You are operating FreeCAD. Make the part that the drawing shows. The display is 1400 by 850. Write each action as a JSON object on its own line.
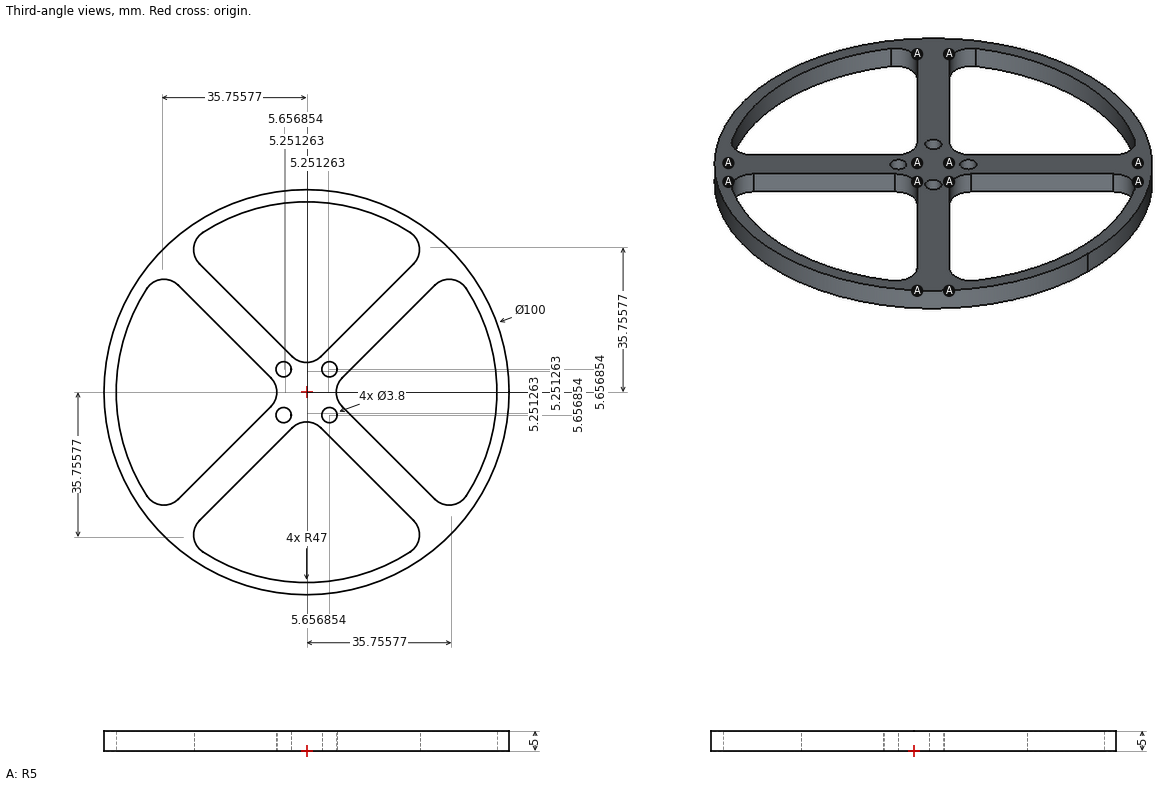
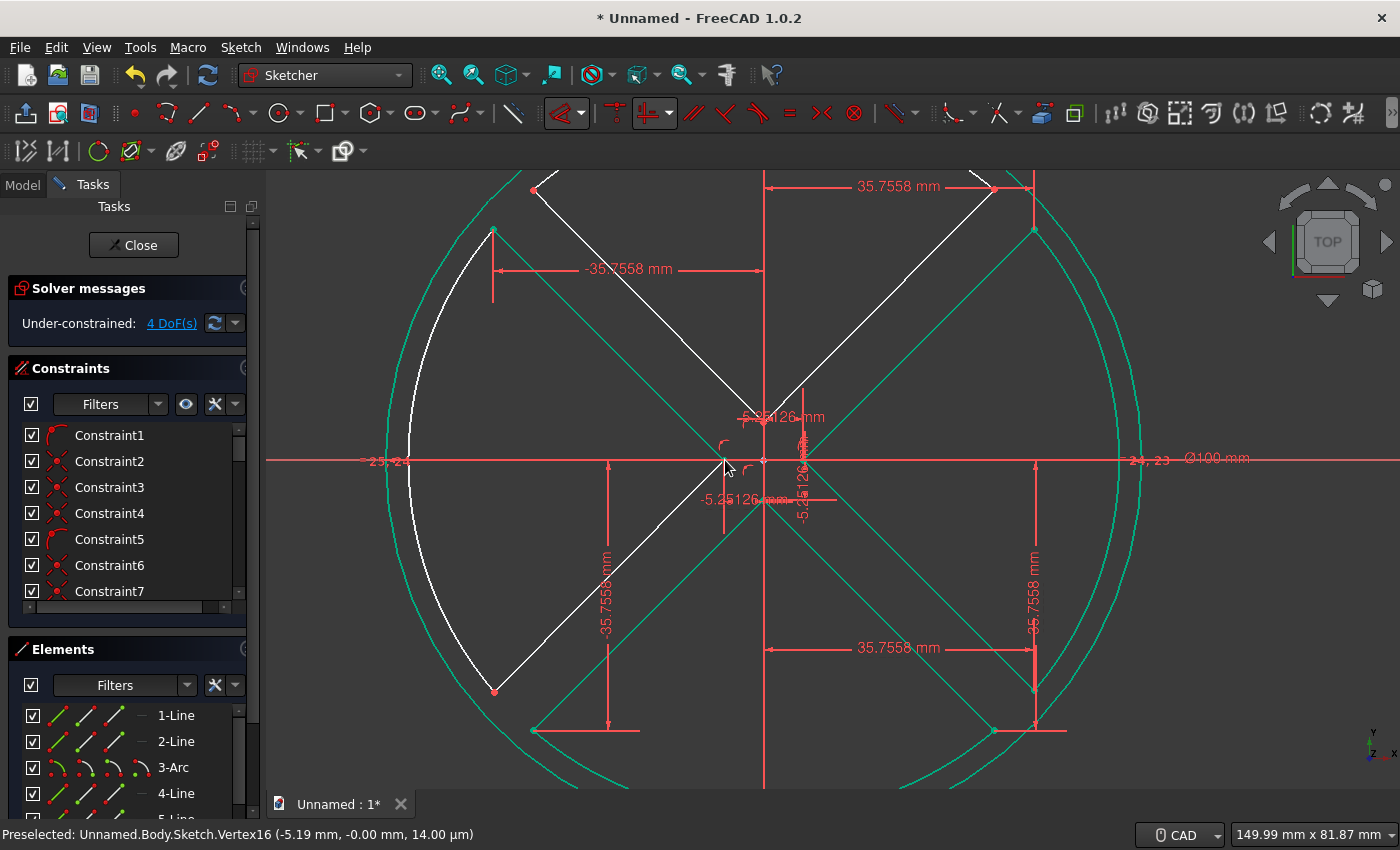
{"action": "left_click", "coordinate": [494, 692]}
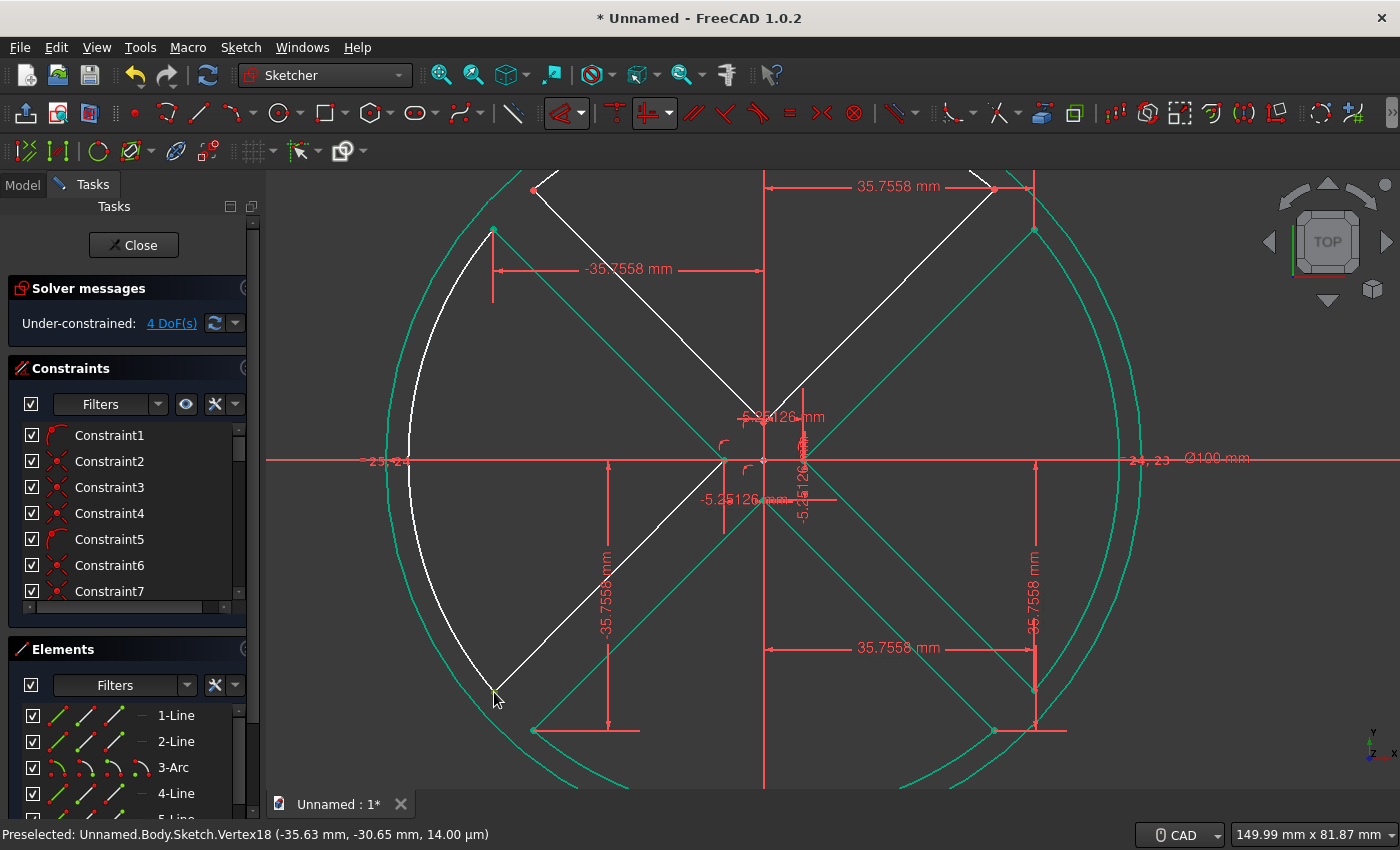
{"action": "key", "text": "l"}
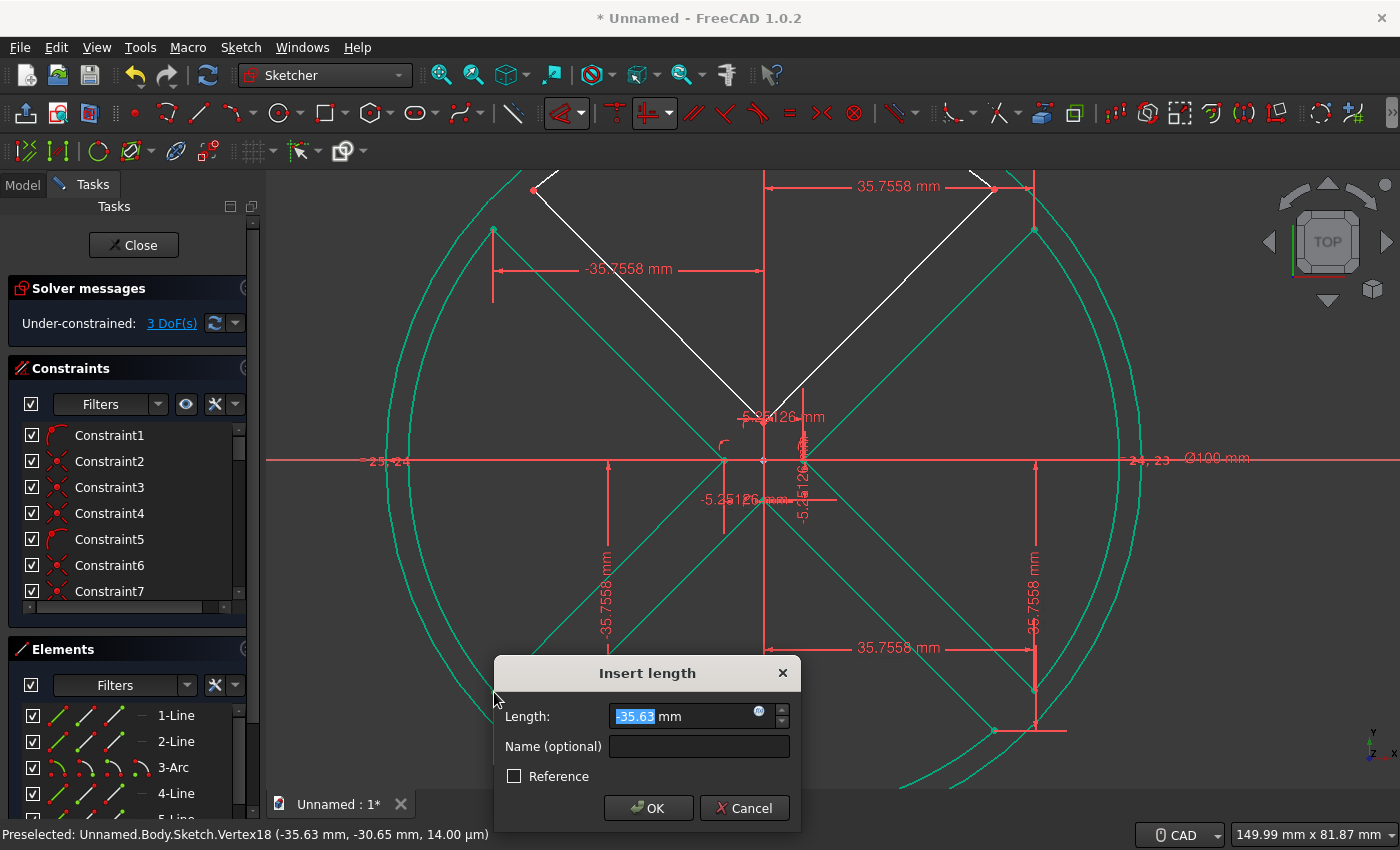
{"action": "type", "text": "-35.75577"}
{"action": "key", "text": "Return"}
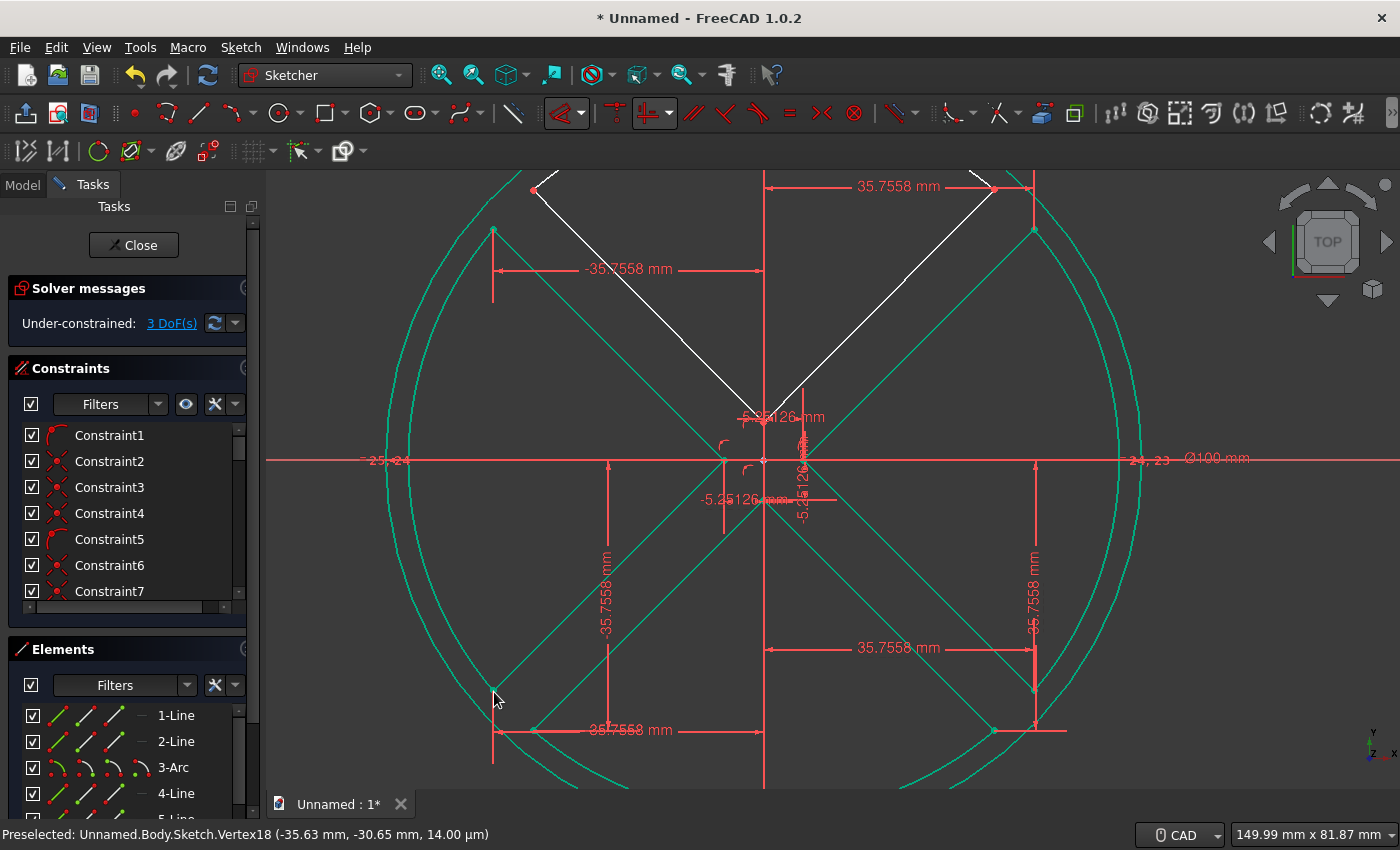
{"action": "scroll", "coordinate": [765, 503], "scroll_direction": "down", "scroll_amount": 3}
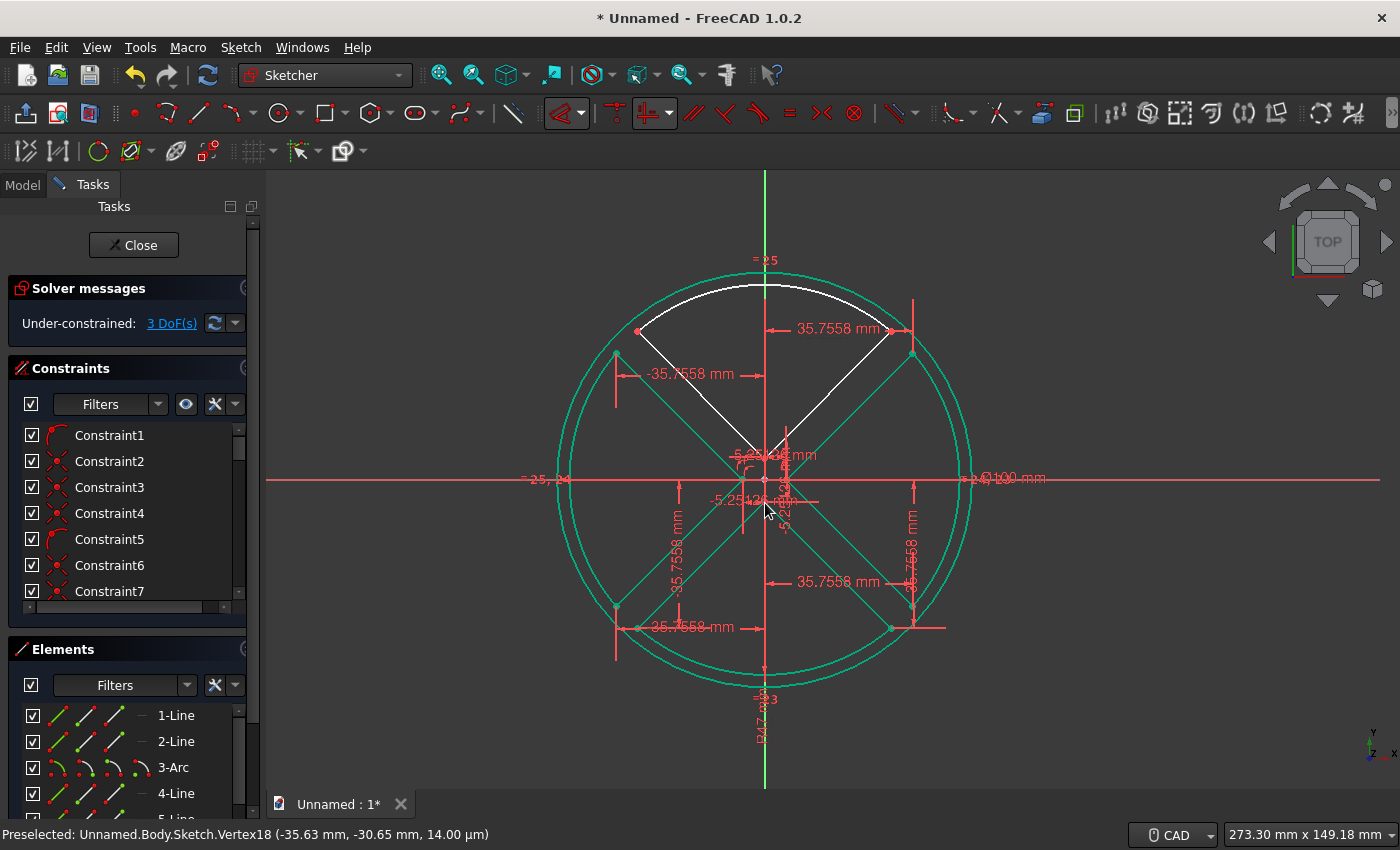
{"action": "left_click", "coordinate": [891, 331]}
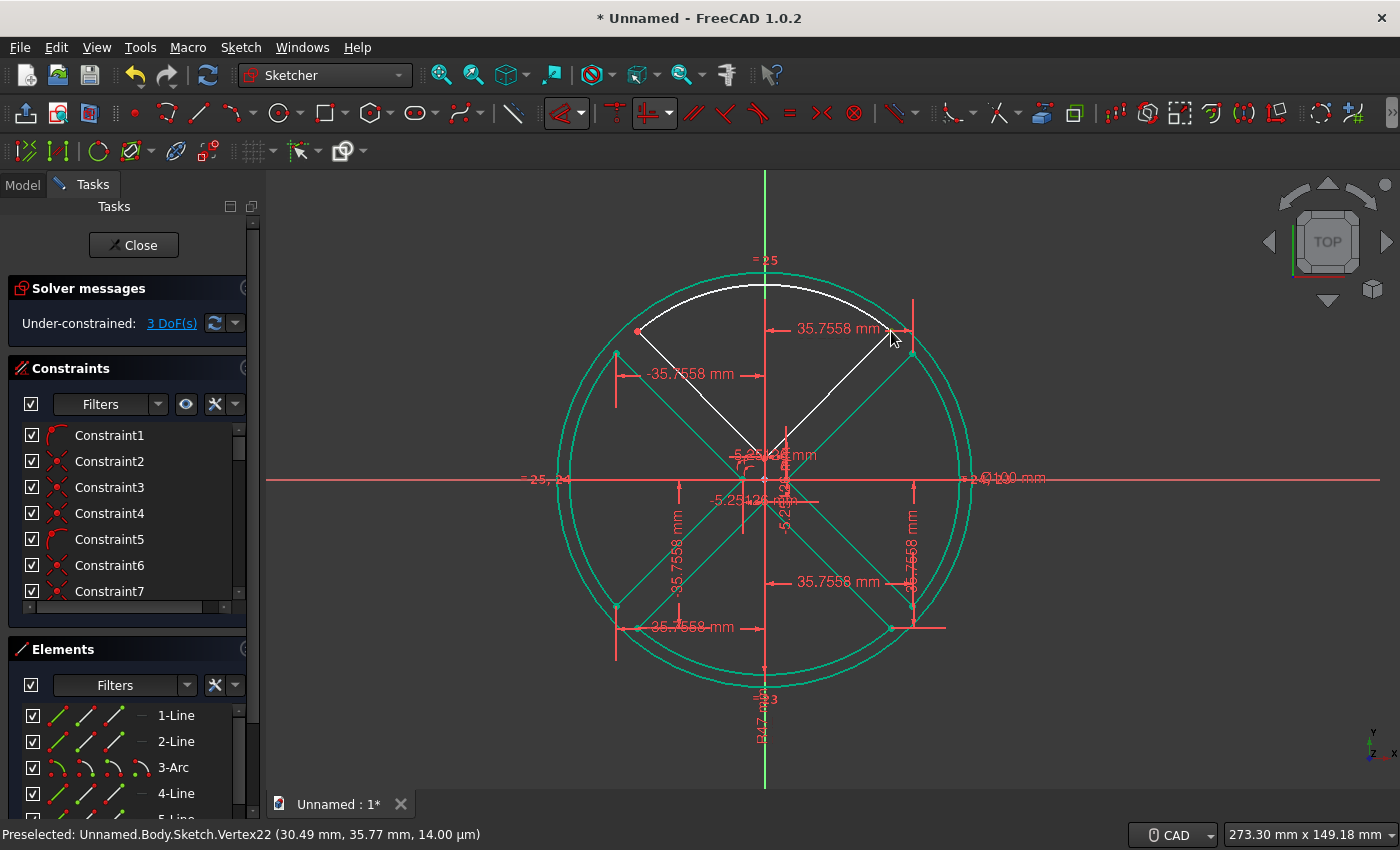
{"action": "left_click", "coordinate": [584, 114]}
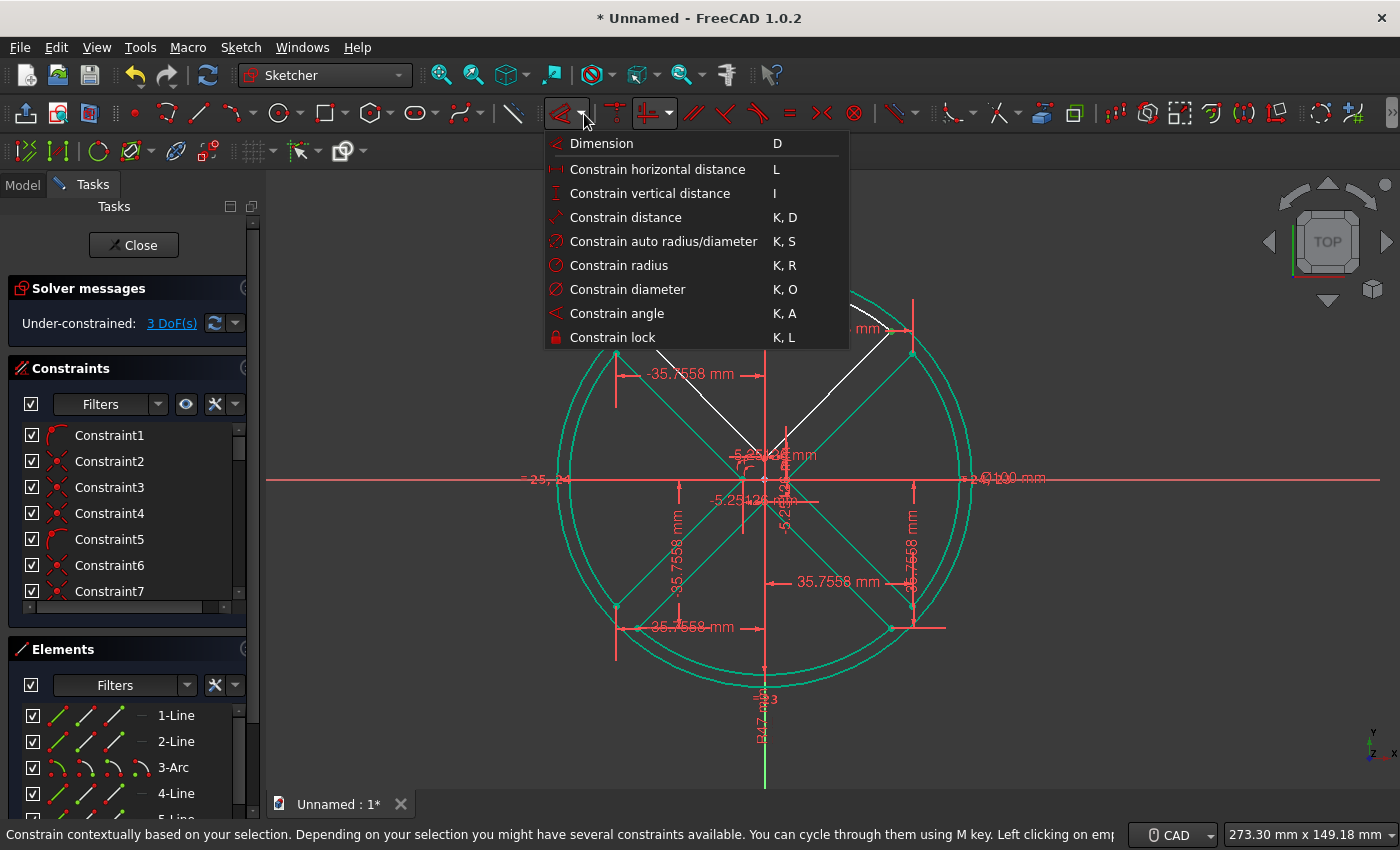
{"action": "left_click", "coordinate": [697, 193]}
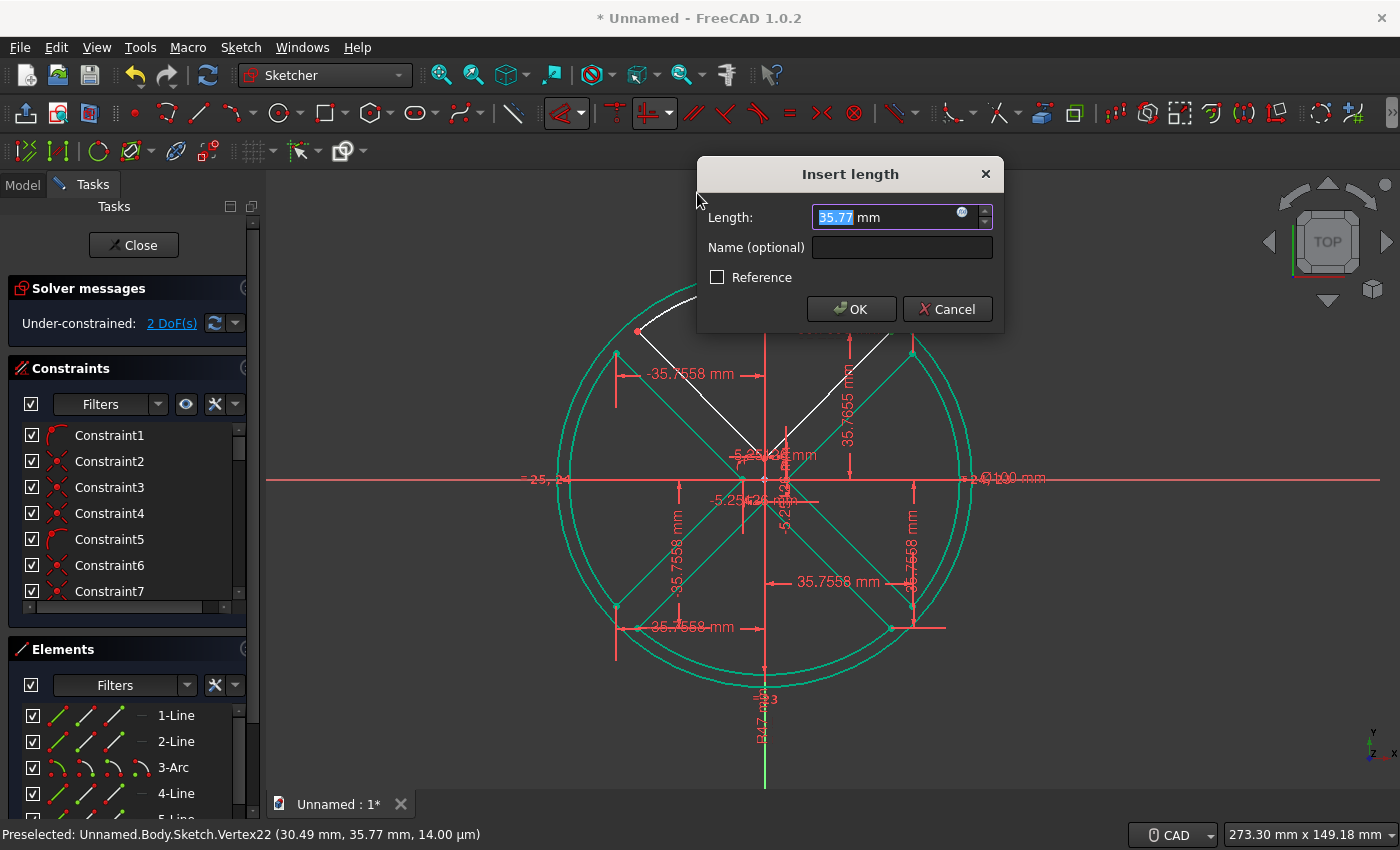
{"action": "type", "text": "35.75577"}
{"action": "key", "text": "Return"}